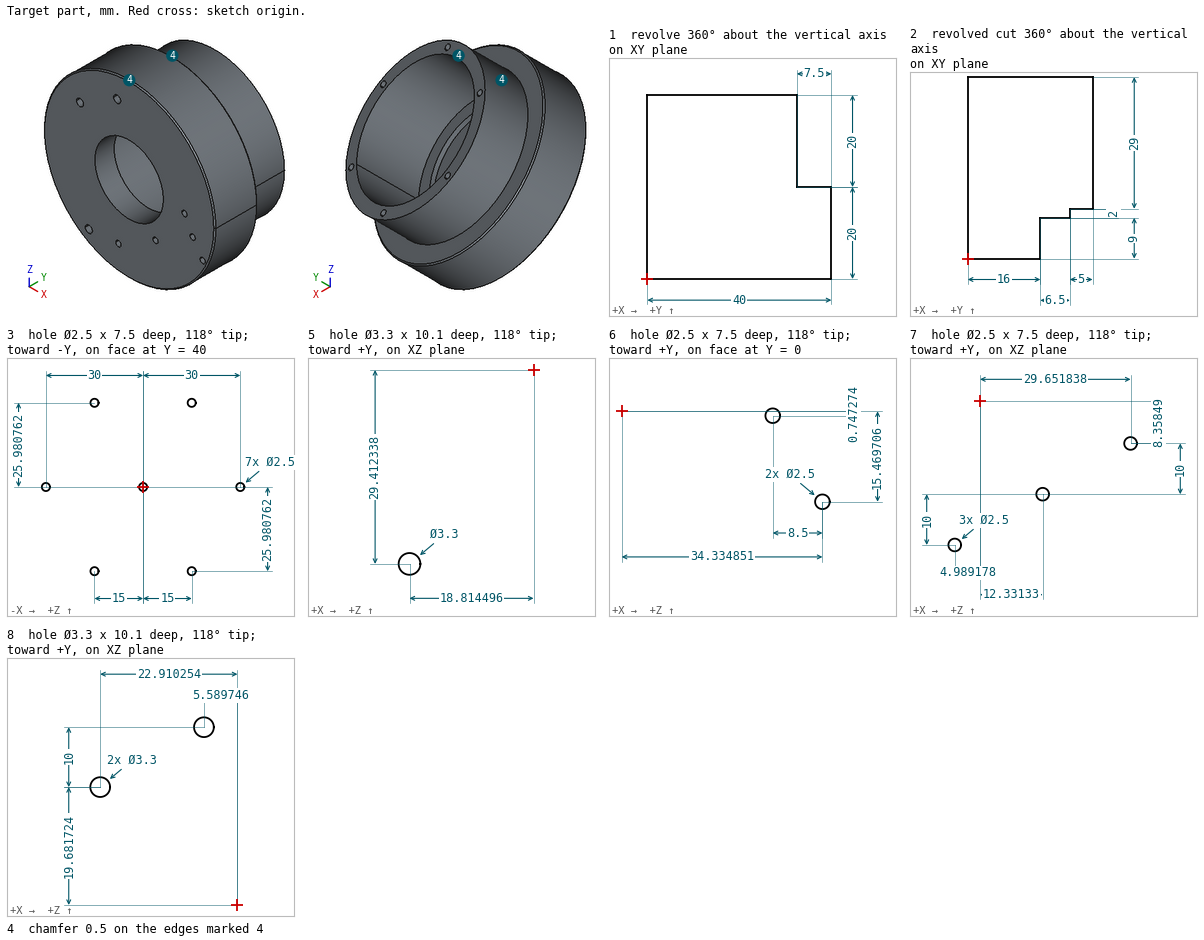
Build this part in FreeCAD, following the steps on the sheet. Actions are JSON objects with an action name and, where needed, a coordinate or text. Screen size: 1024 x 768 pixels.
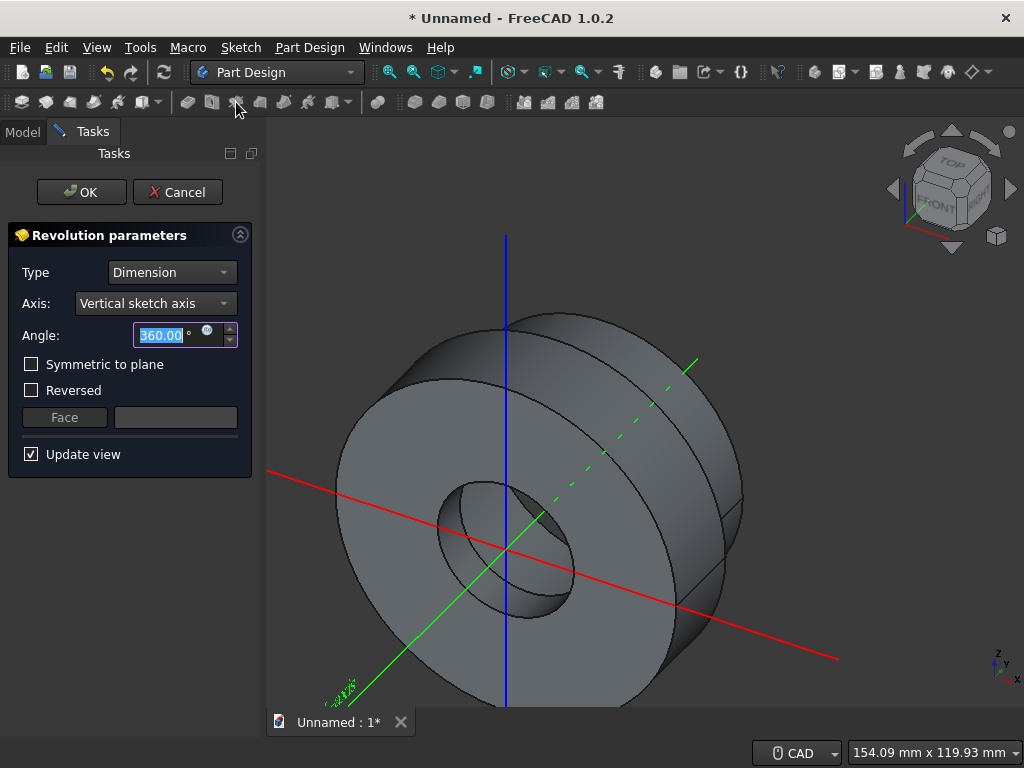
{"action": "left_click", "coordinate": [82, 192]}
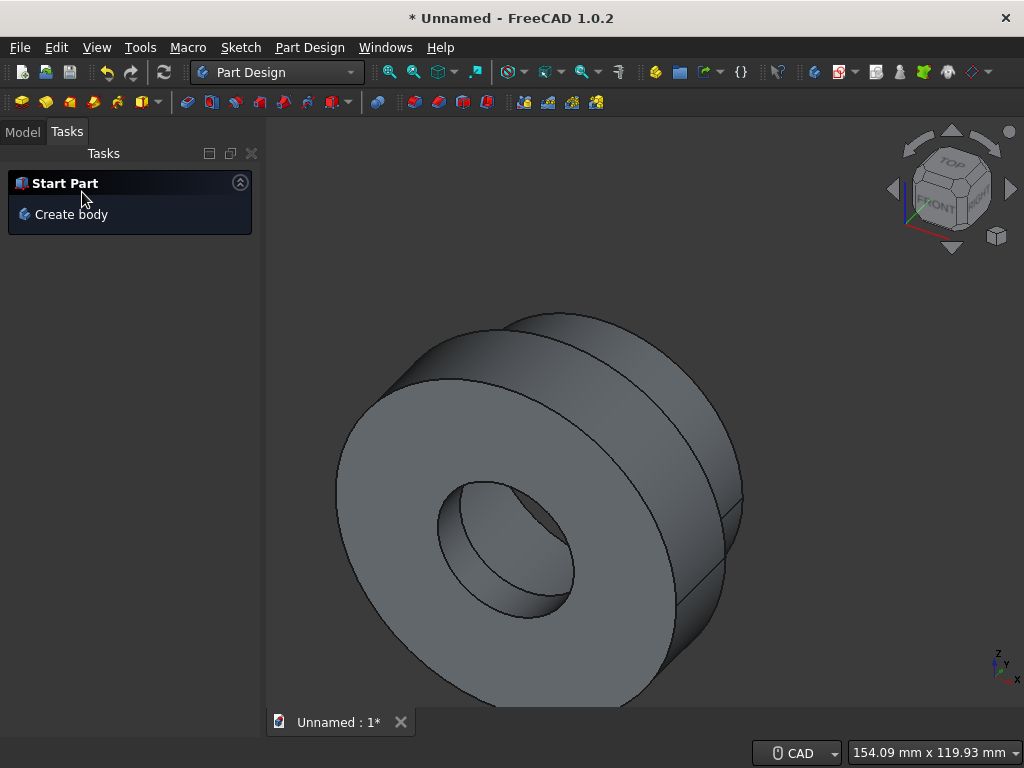
{"action": "left_click", "coordinate": [390, 72]}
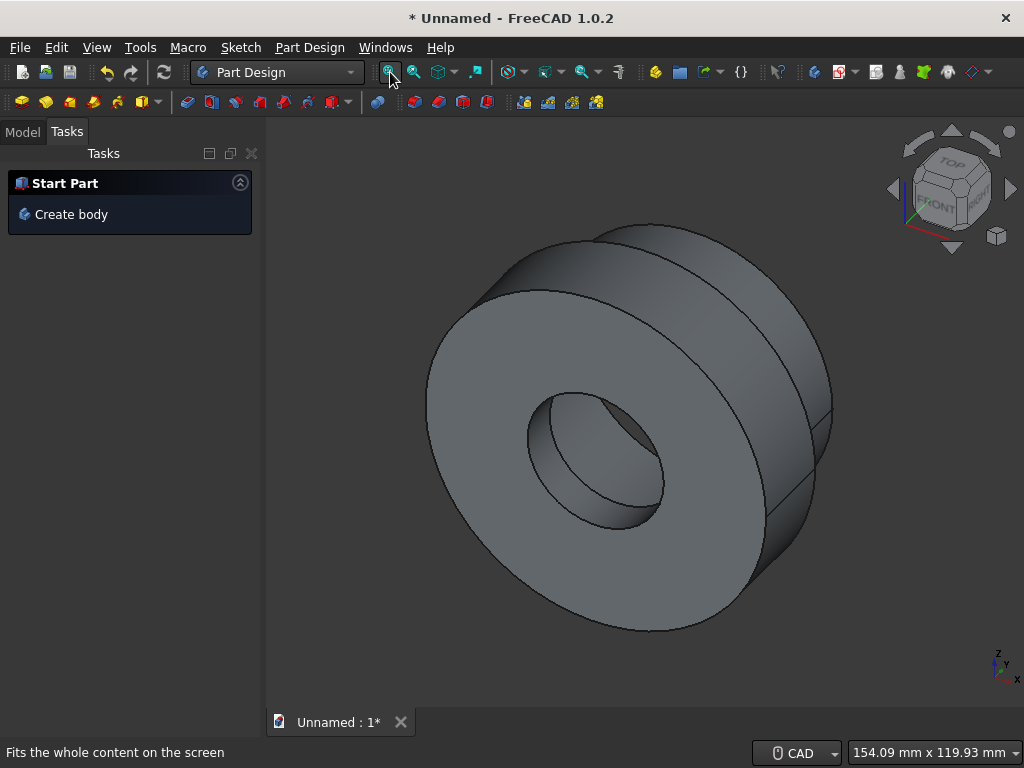
{"action": "key", "text": "4"}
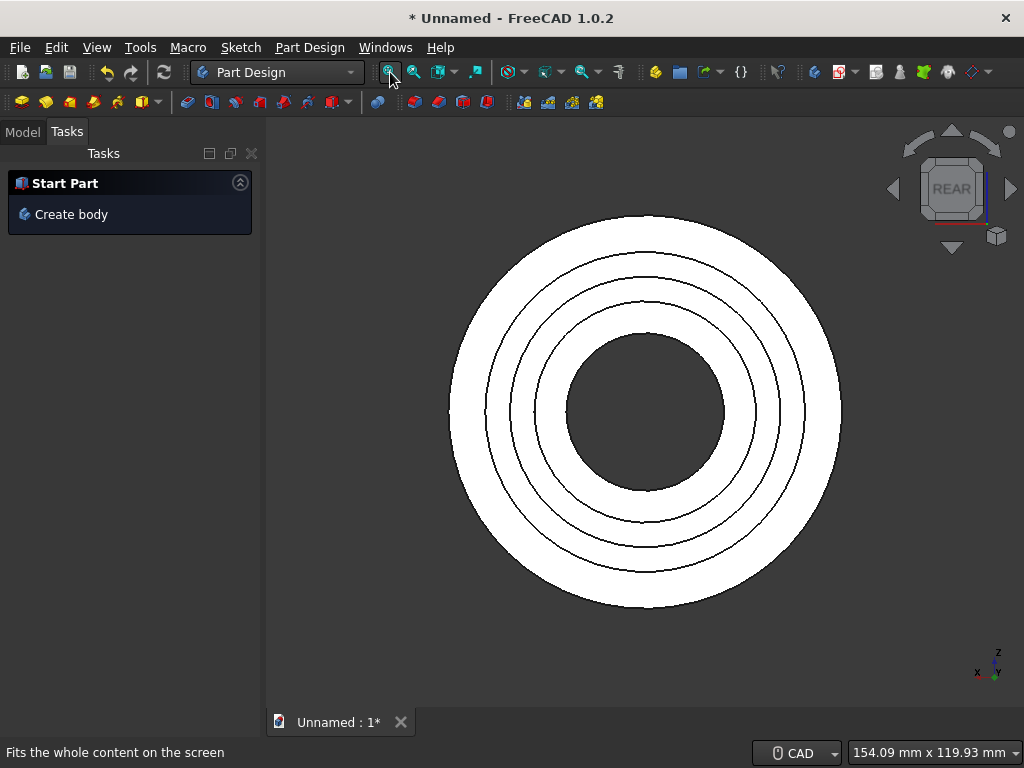
{"action": "left_click", "coordinate": [599, 548]}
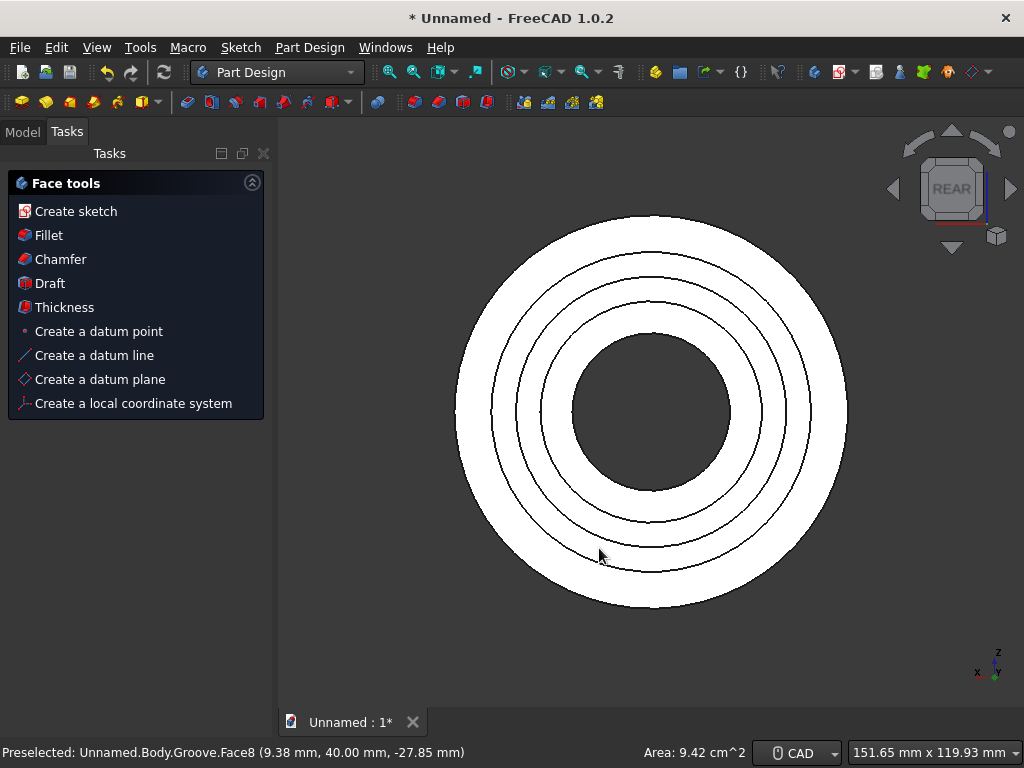
{"action": "left_click", "coordinate": [840, 72]}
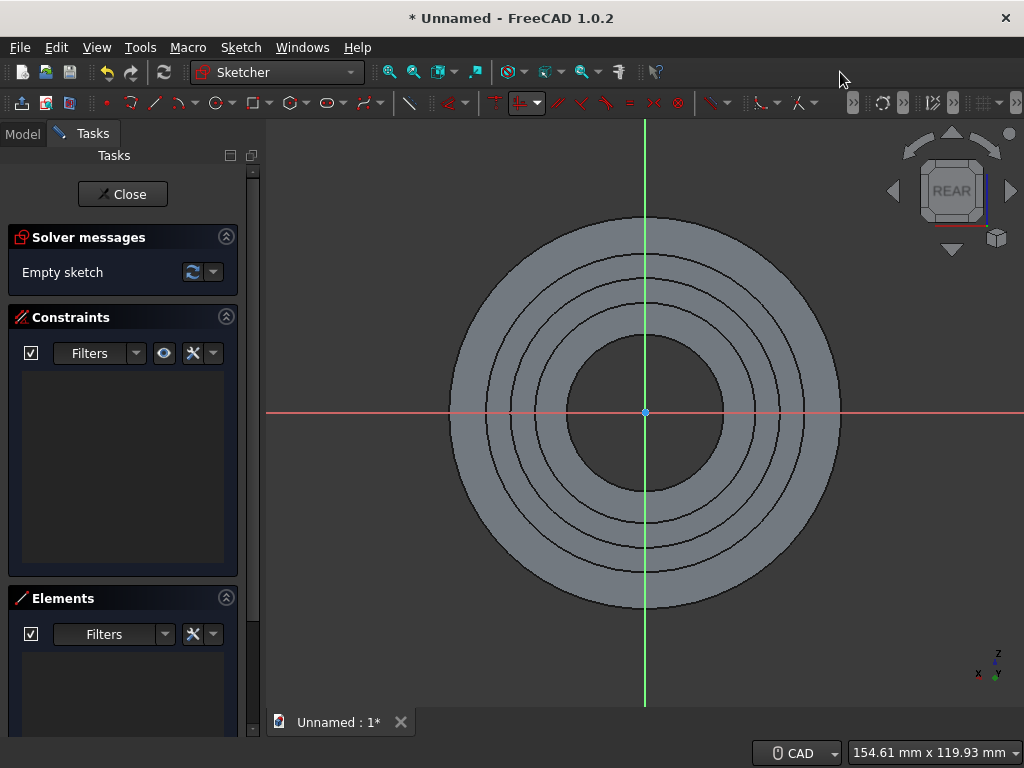
{"action": "left_click", "coordinate": [216, 104]}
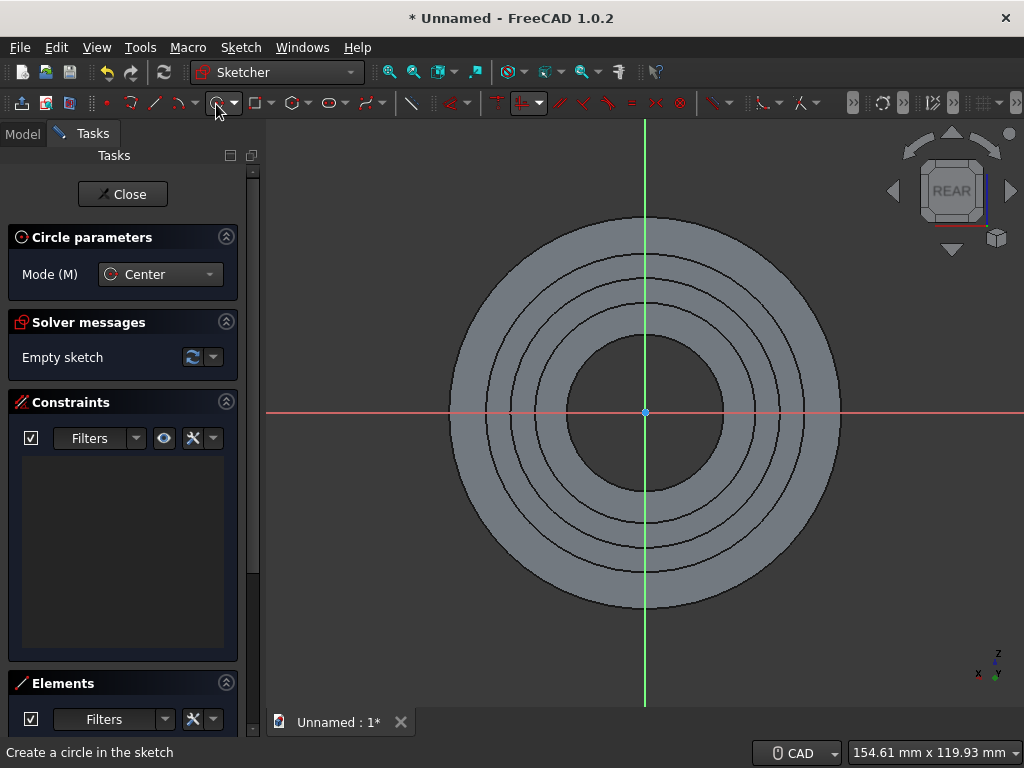
{"action": "scroll", "coordinate": [792, 413], "scroll_direction": "up", "scroll_amount": 7}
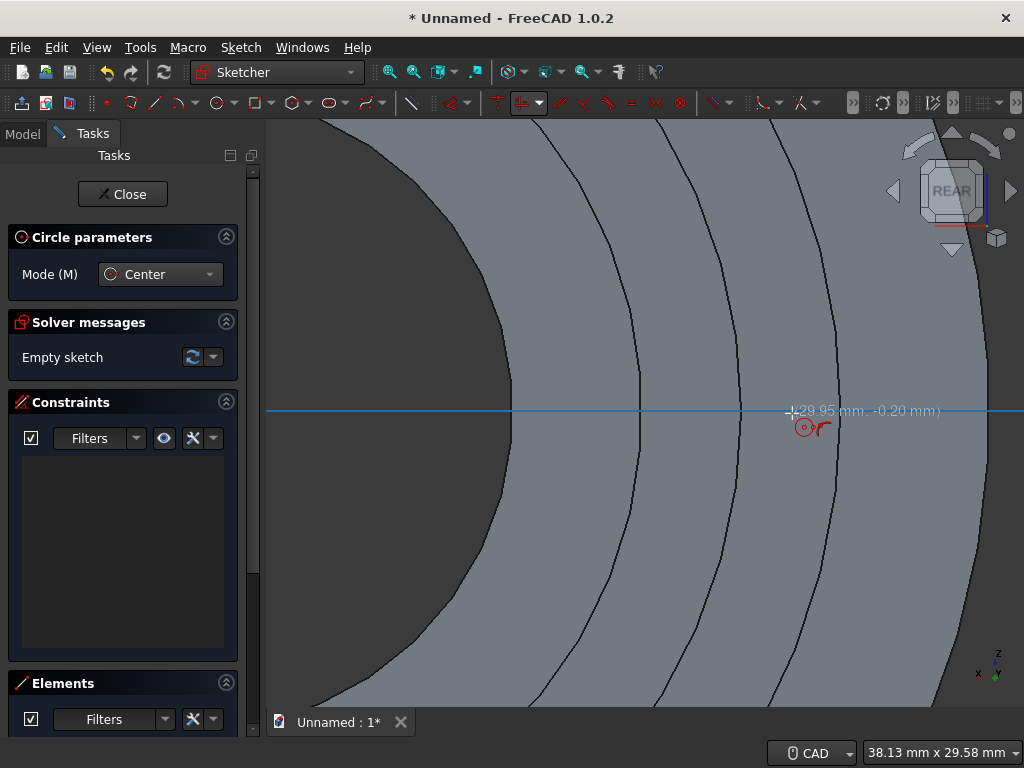
{"action": "scroll", "coordinate": [741, 414], "scroll_direction": "down", "scroll_amount": 6}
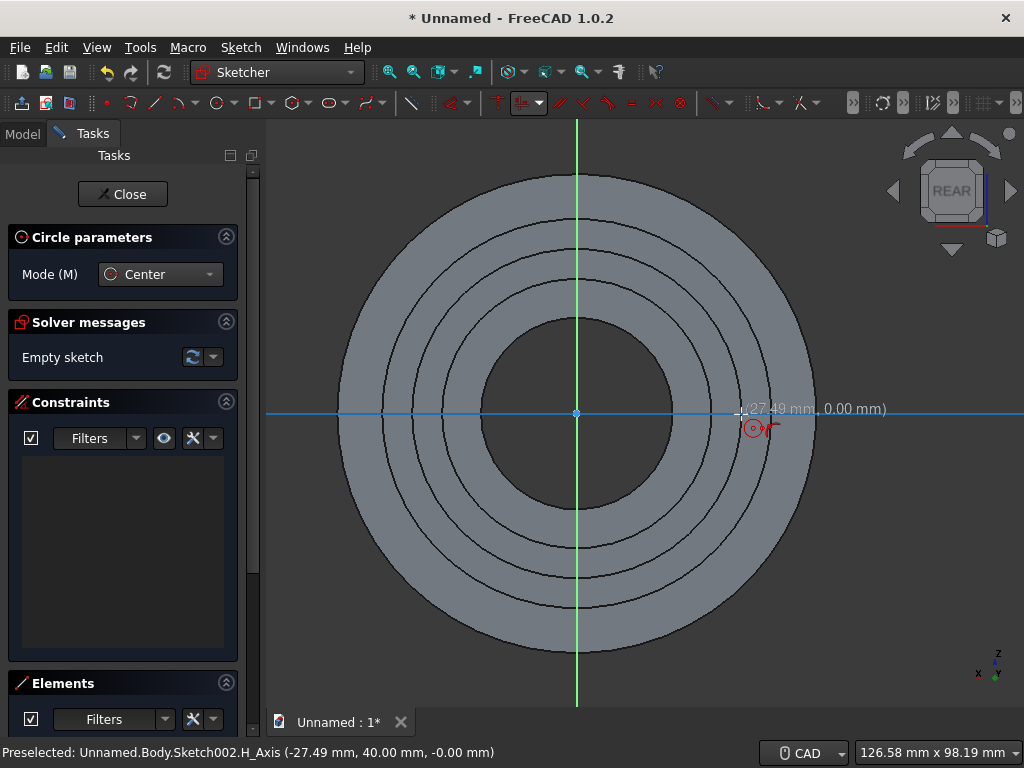
{"action": "left_click", "coordinate": [756, 414]}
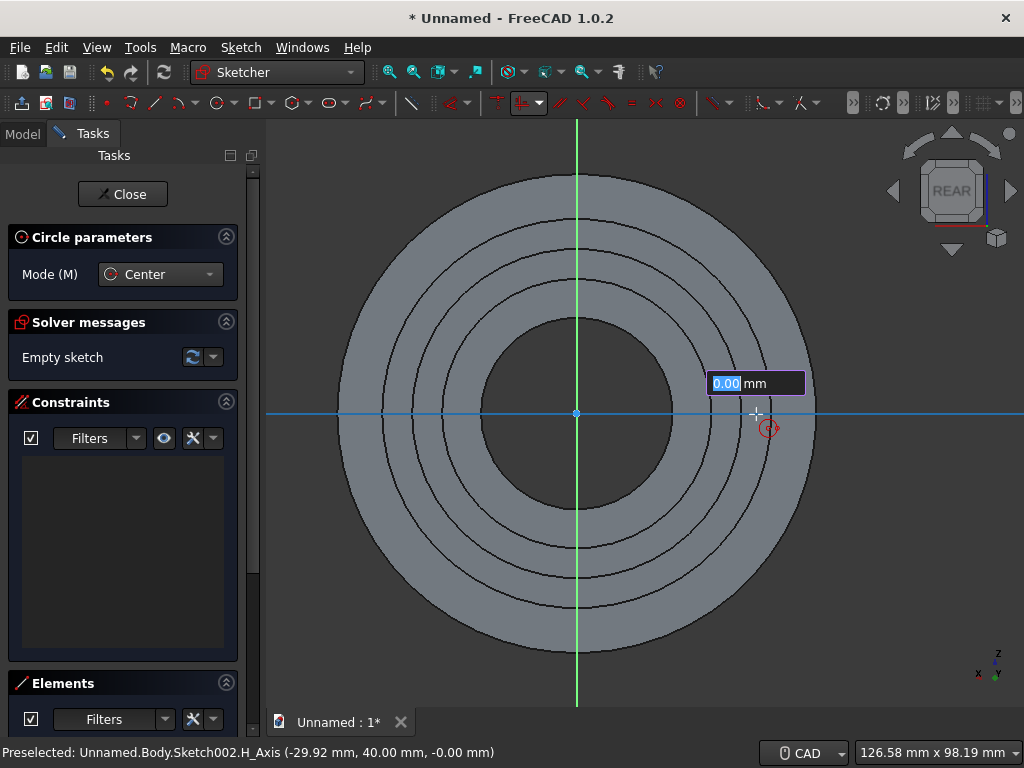
{"action": "scroll", "coordinate": [754, 421], "scroll_direction": "up", "scroll_amount": 5}
{"action": "mouse_move", "coordinate": [753, 419]}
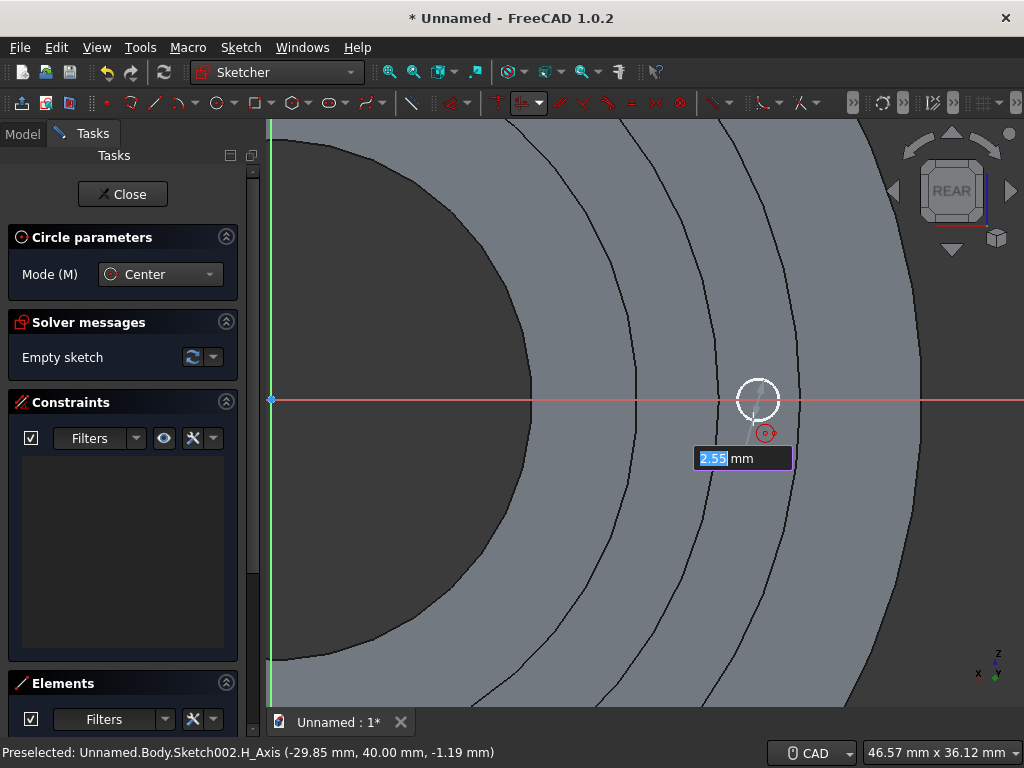
{"action": "type", "text": "2.5"}
{"action": "key", "text": "Return"}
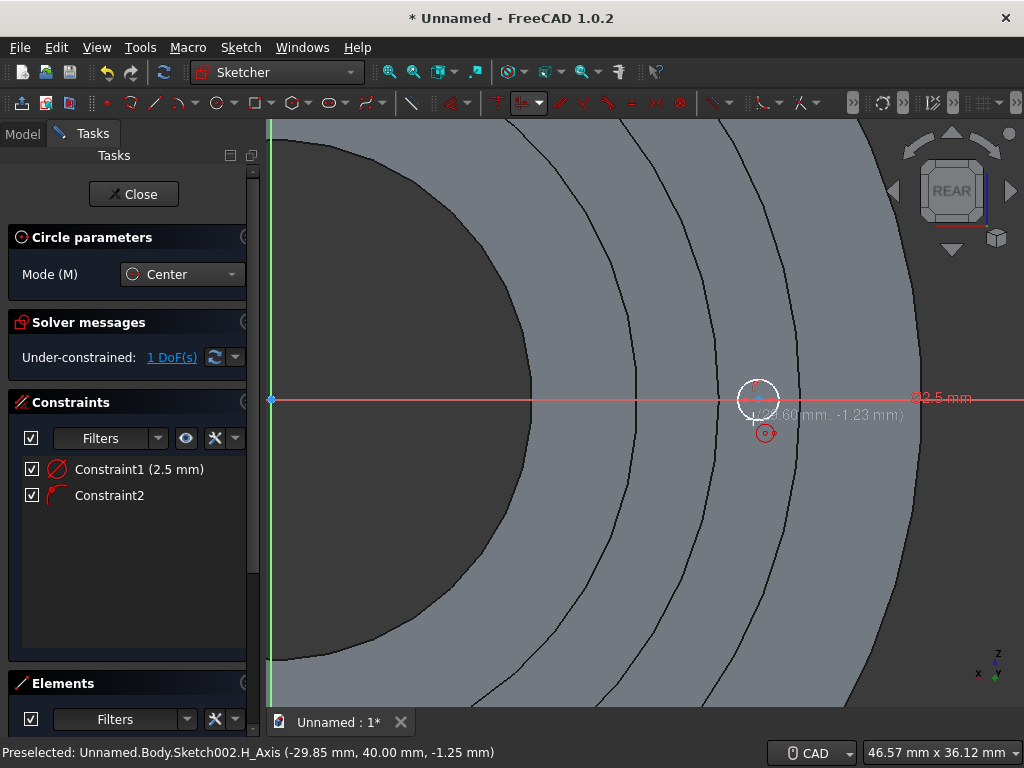
{"action": "scroll", "coordinate": [754, 421], "scroll_direction": "down", "scroll_amount": 5}